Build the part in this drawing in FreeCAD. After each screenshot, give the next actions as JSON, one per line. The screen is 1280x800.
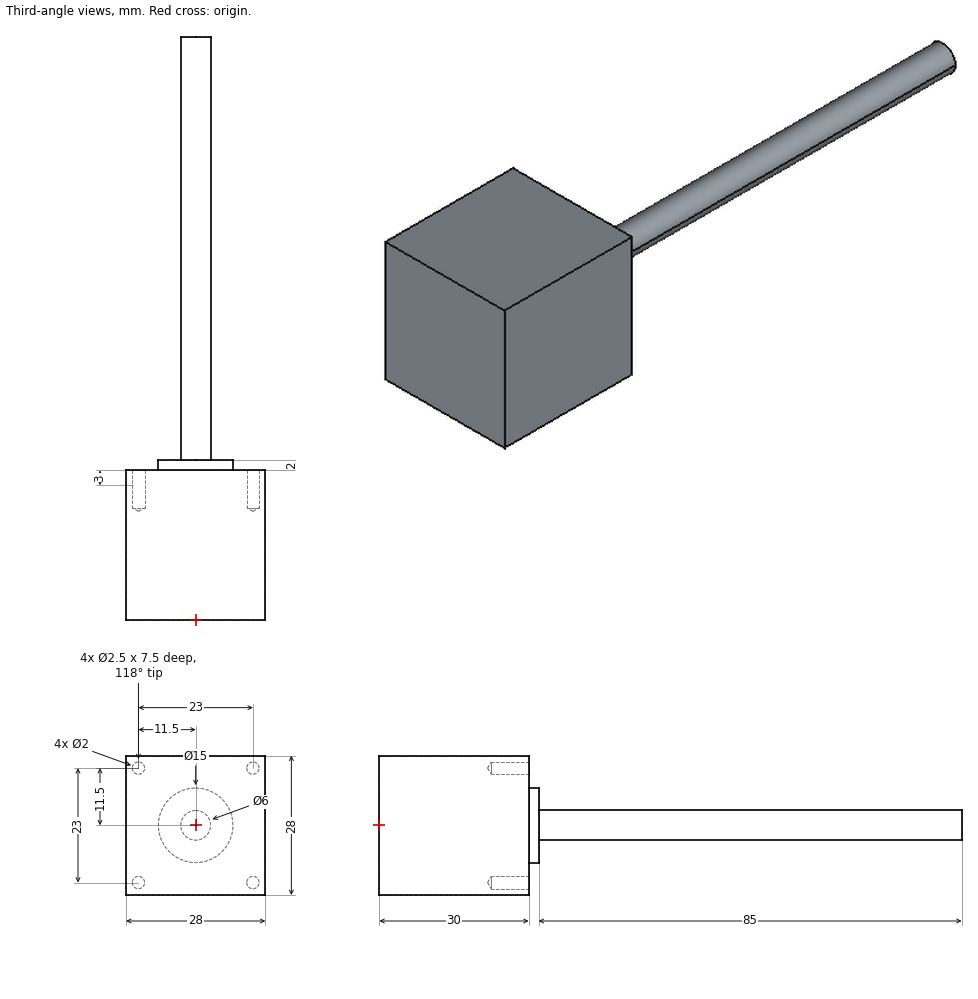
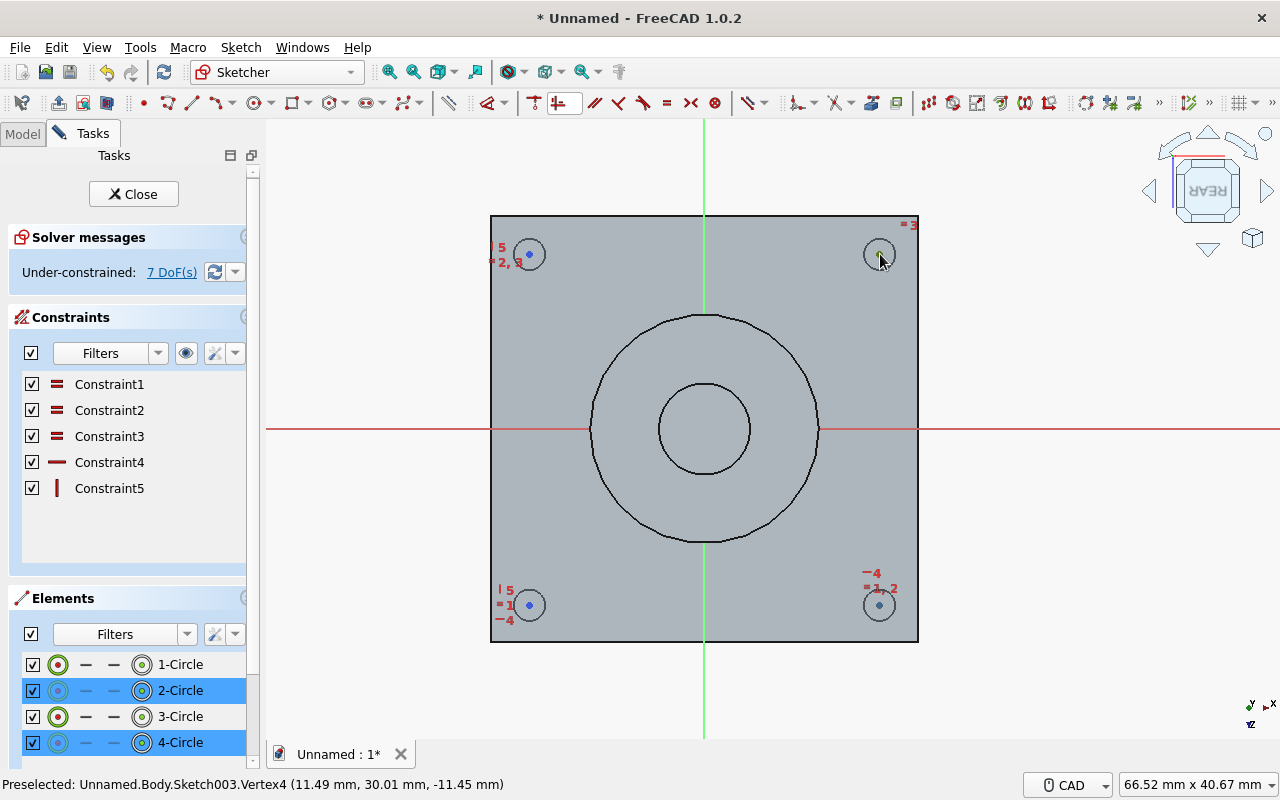
{"action": "key", "text": "v"}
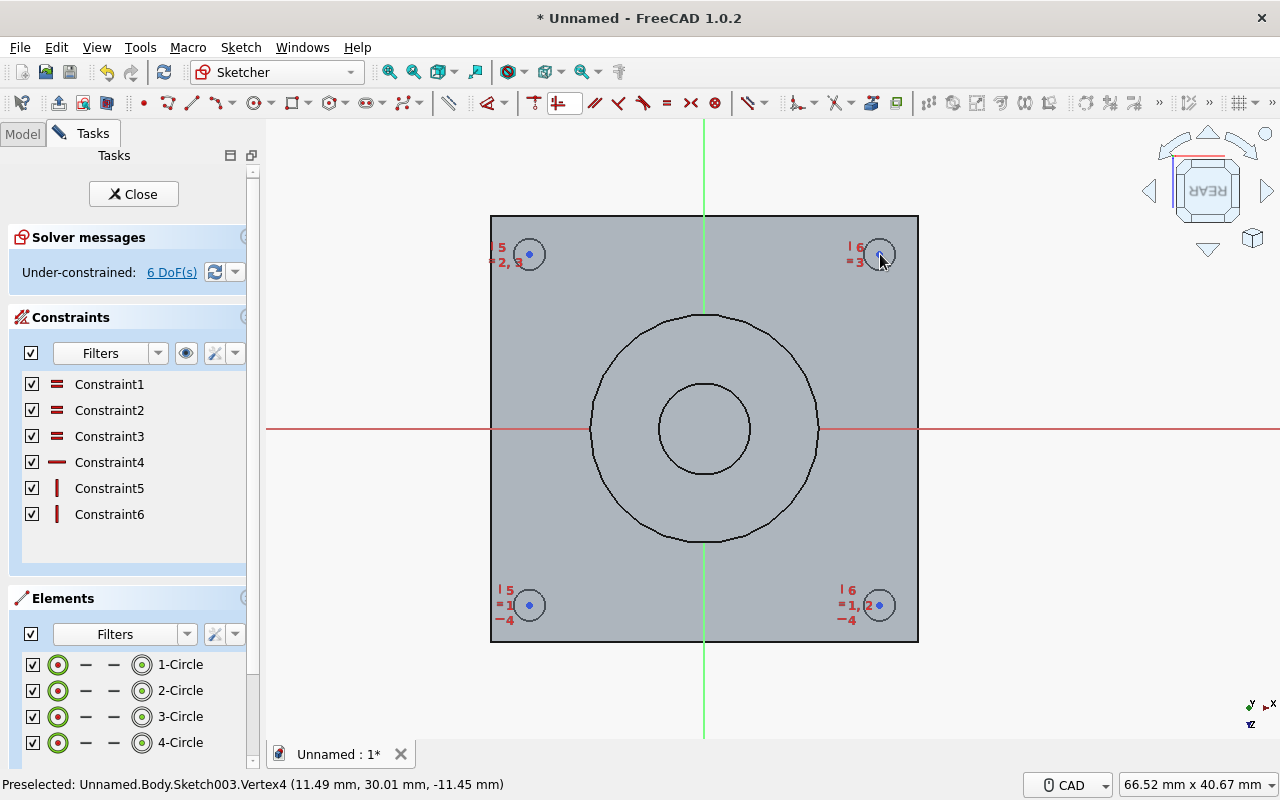
{"action": "left_click", "coordinate": [529, 254]}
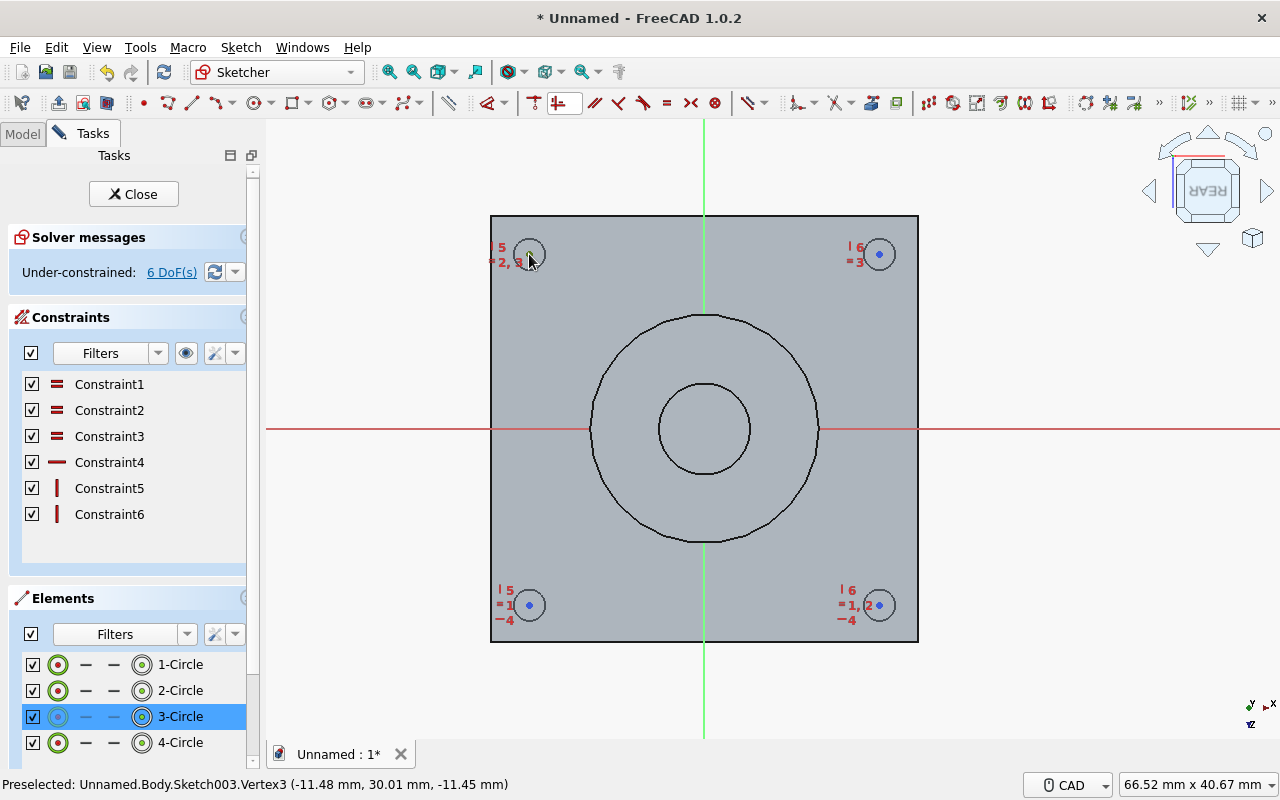
{"action": "left_click", "coordinate": [880, 254]}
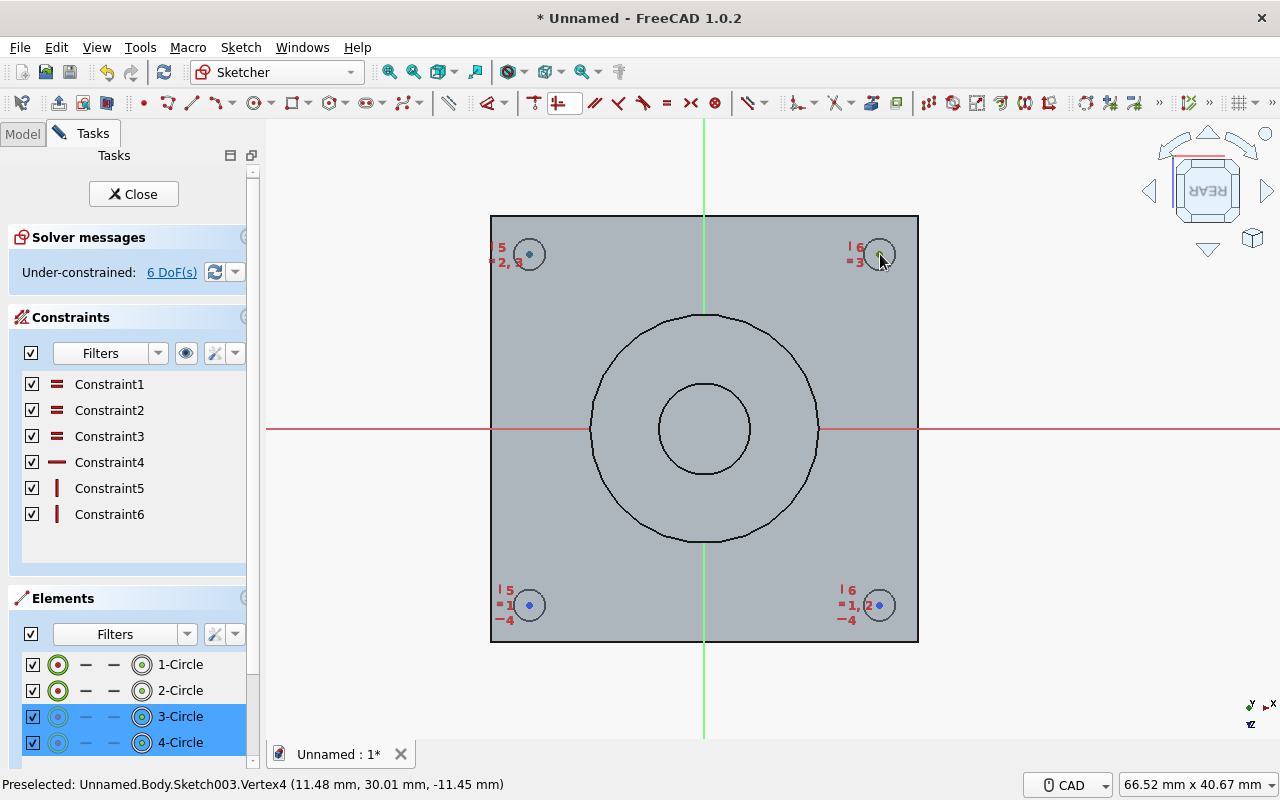
{"action": "left_click", "coordinate": [576, 104]}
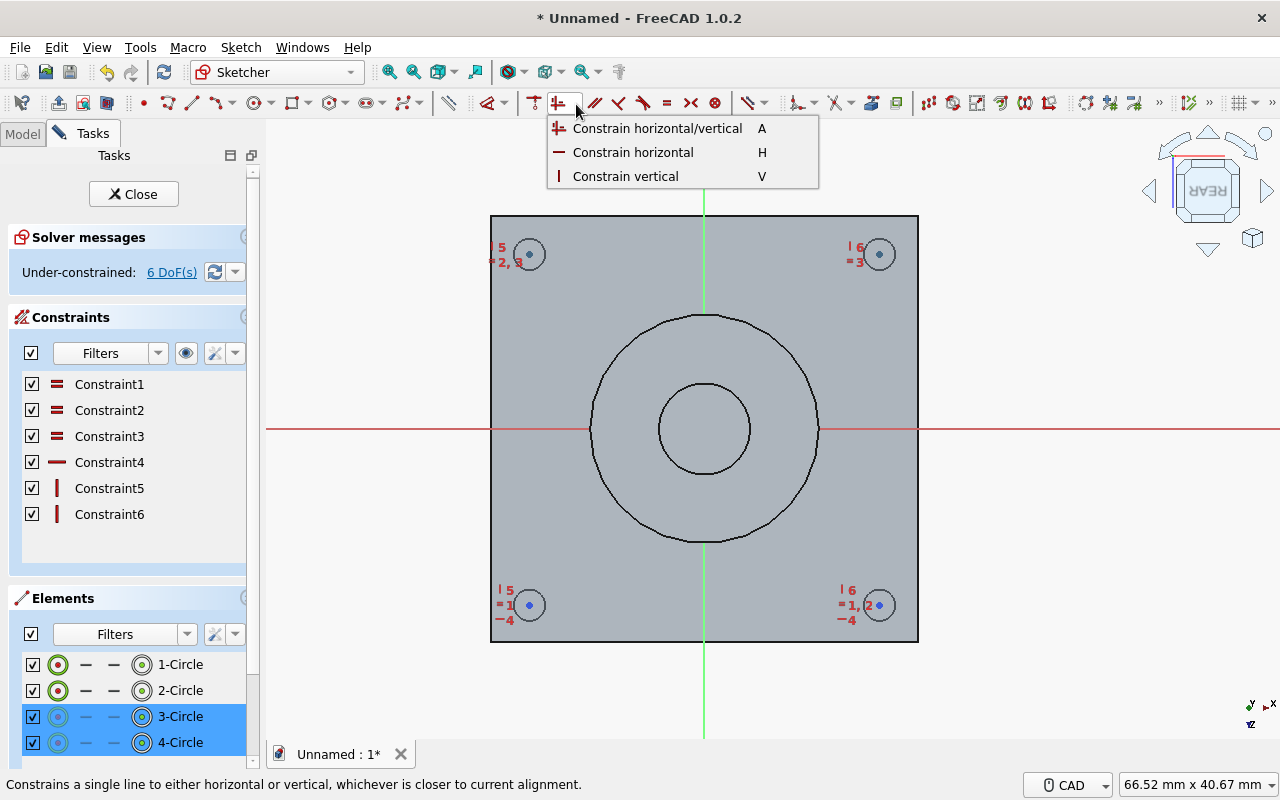
{"action": "left_click", "coordinate": [683, 152]}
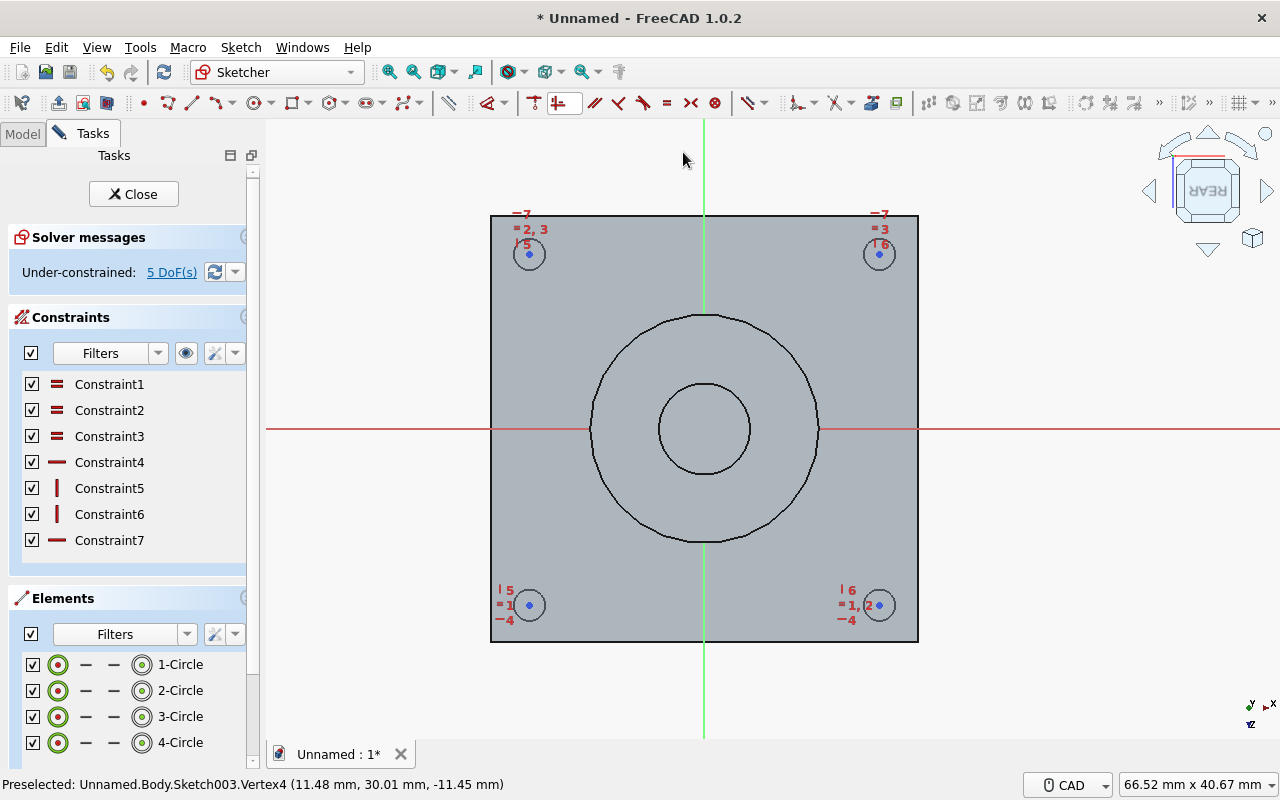
{"action": "left_click", "coordinate": [488, 104]}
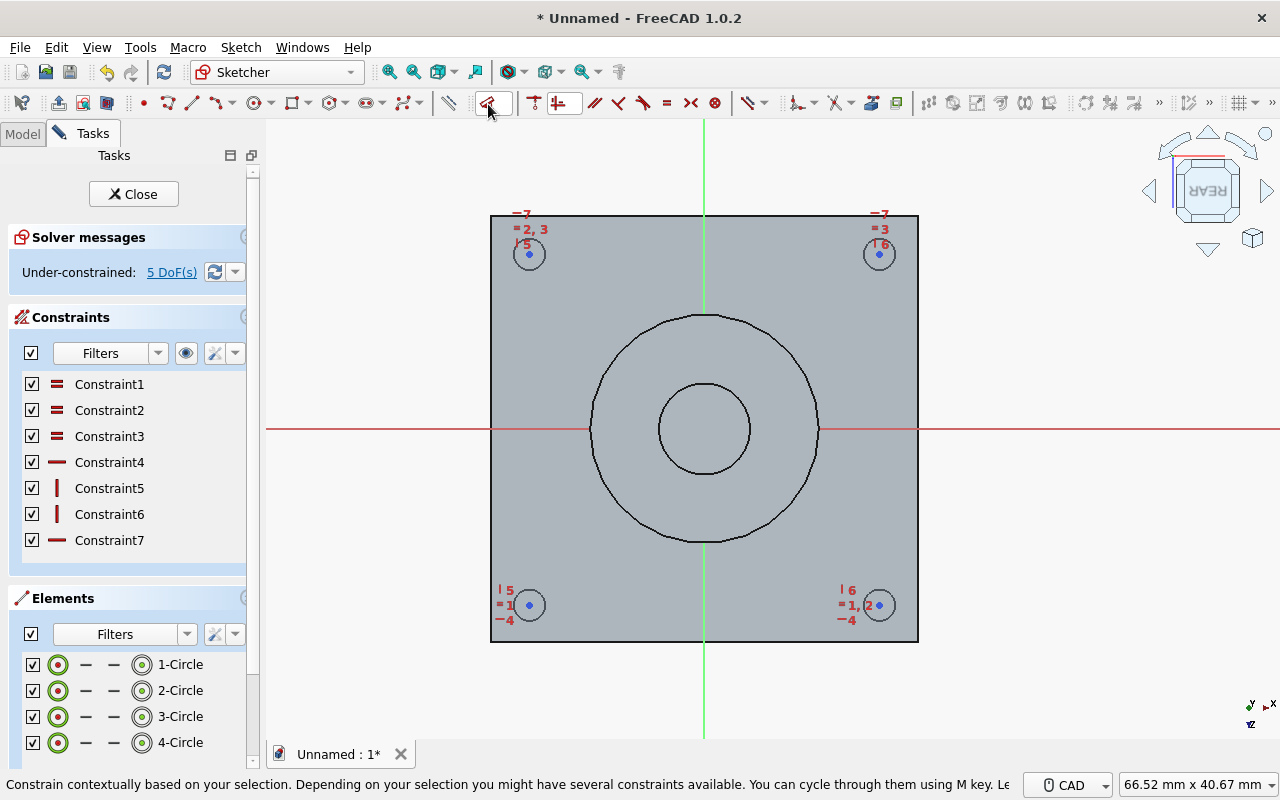
{"action": "scroll", "coordinate": [540, 594], "scroll_direction": "up", "scroll_amount": 2}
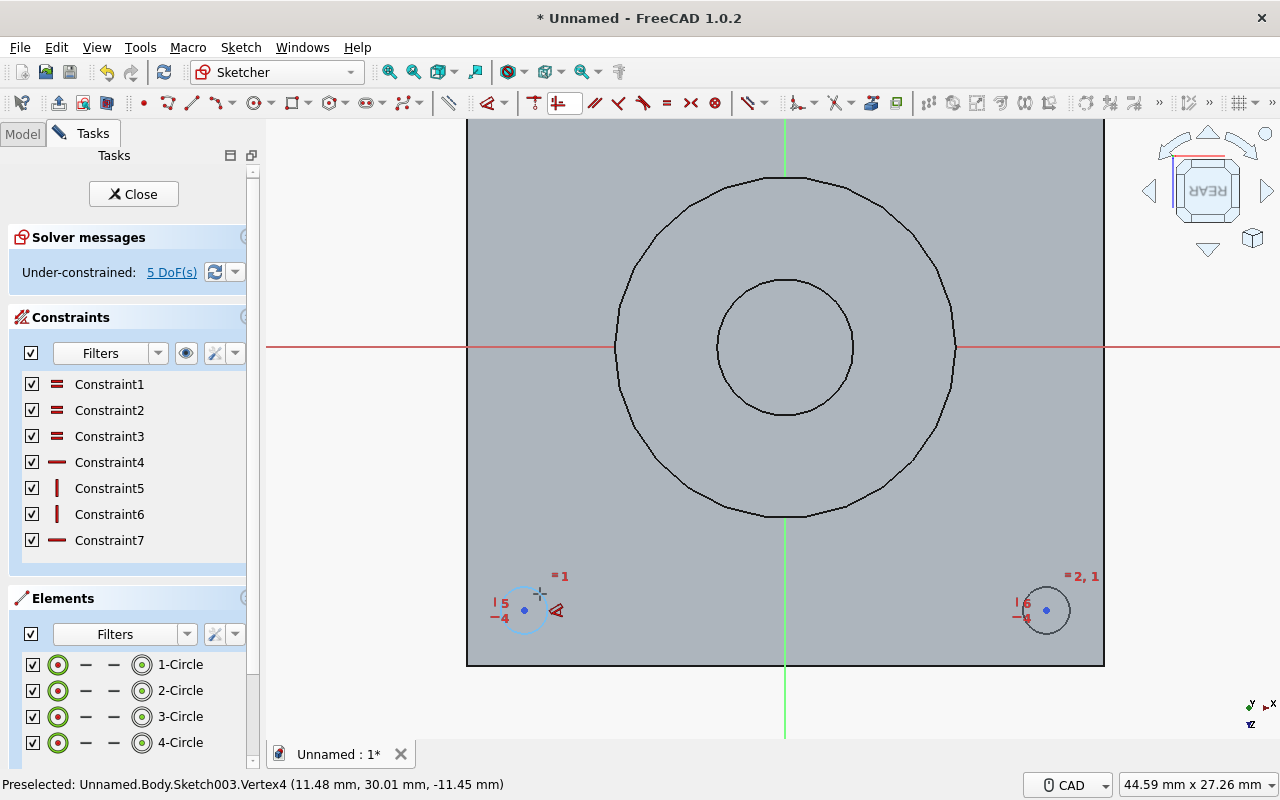
{"action": "left_click", "coordinate": [541, 594]}
{"action": "left_click", "coordinate": [564, 572]}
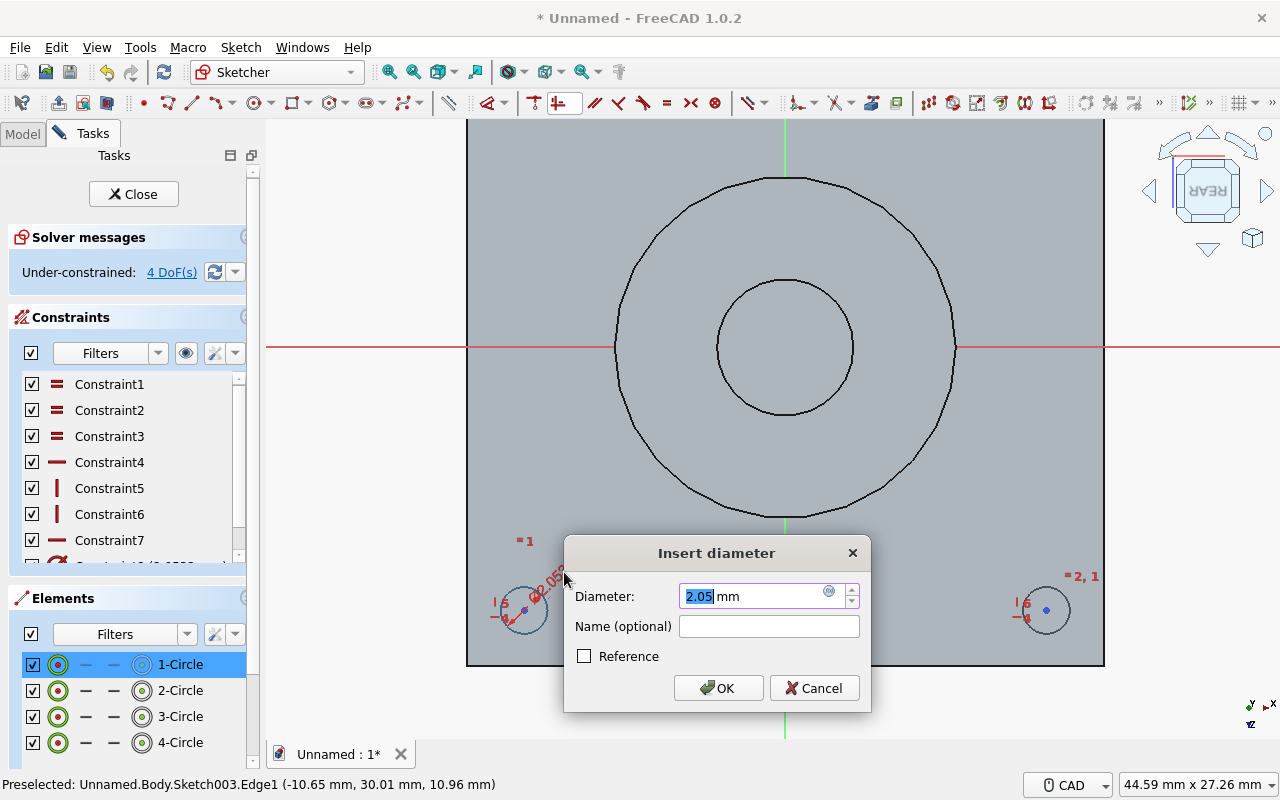
{"action": "type", "text": "2"}
{"action": "key", "text": "Return"}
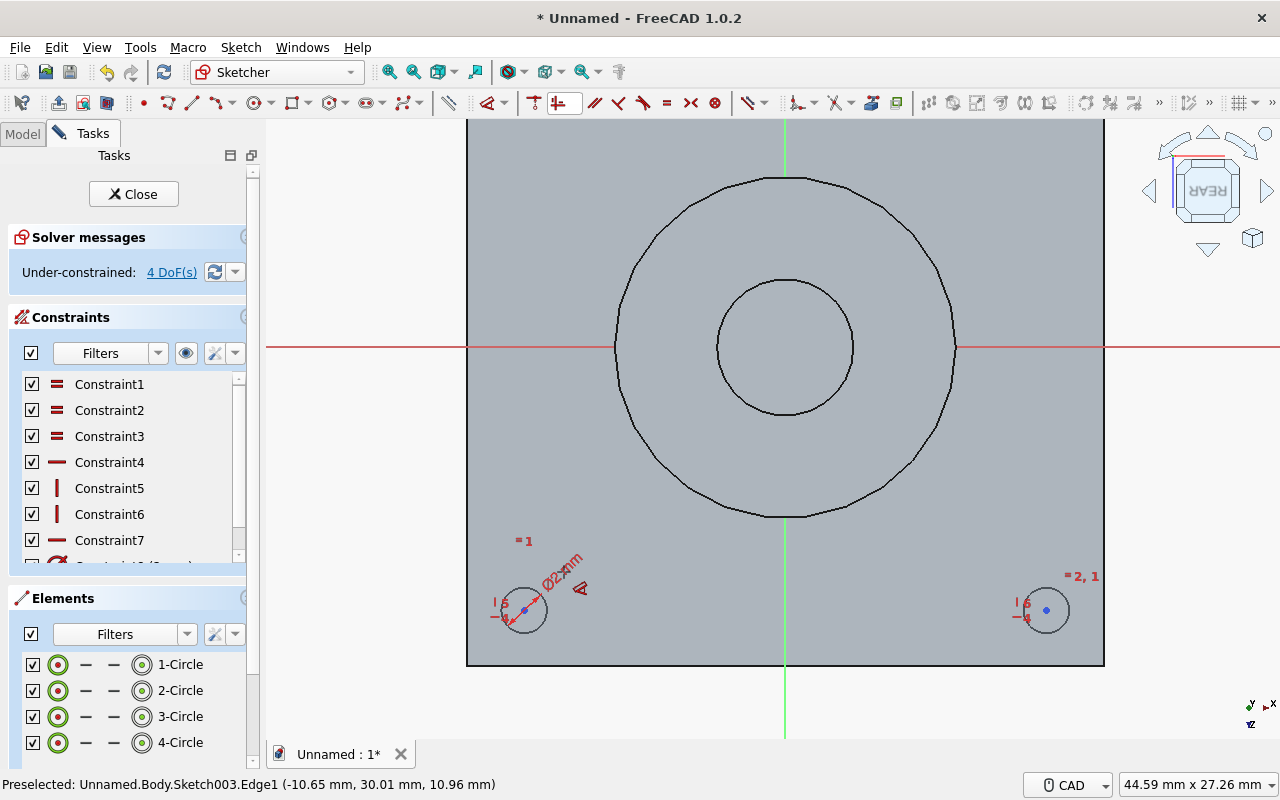
{"action": "left_click", "coordinate": [524, 610]}